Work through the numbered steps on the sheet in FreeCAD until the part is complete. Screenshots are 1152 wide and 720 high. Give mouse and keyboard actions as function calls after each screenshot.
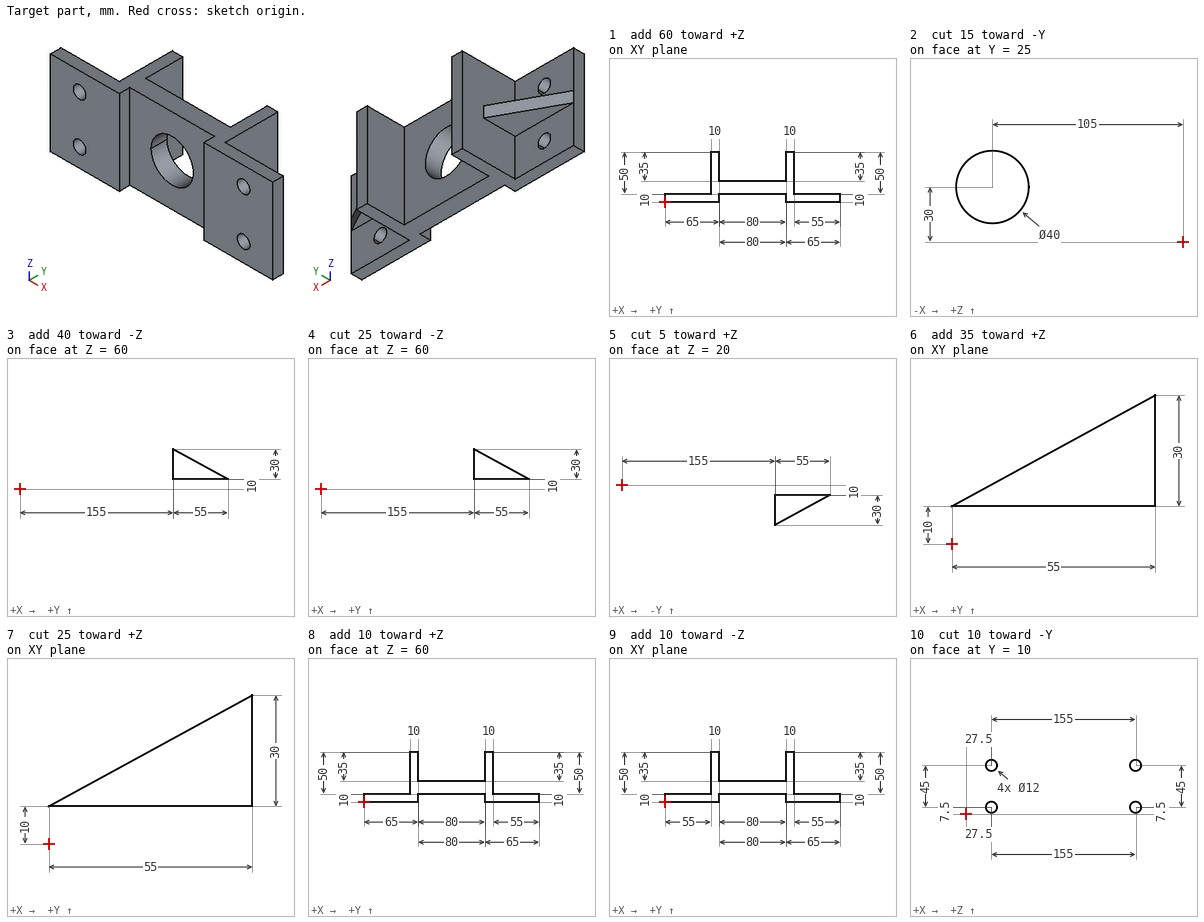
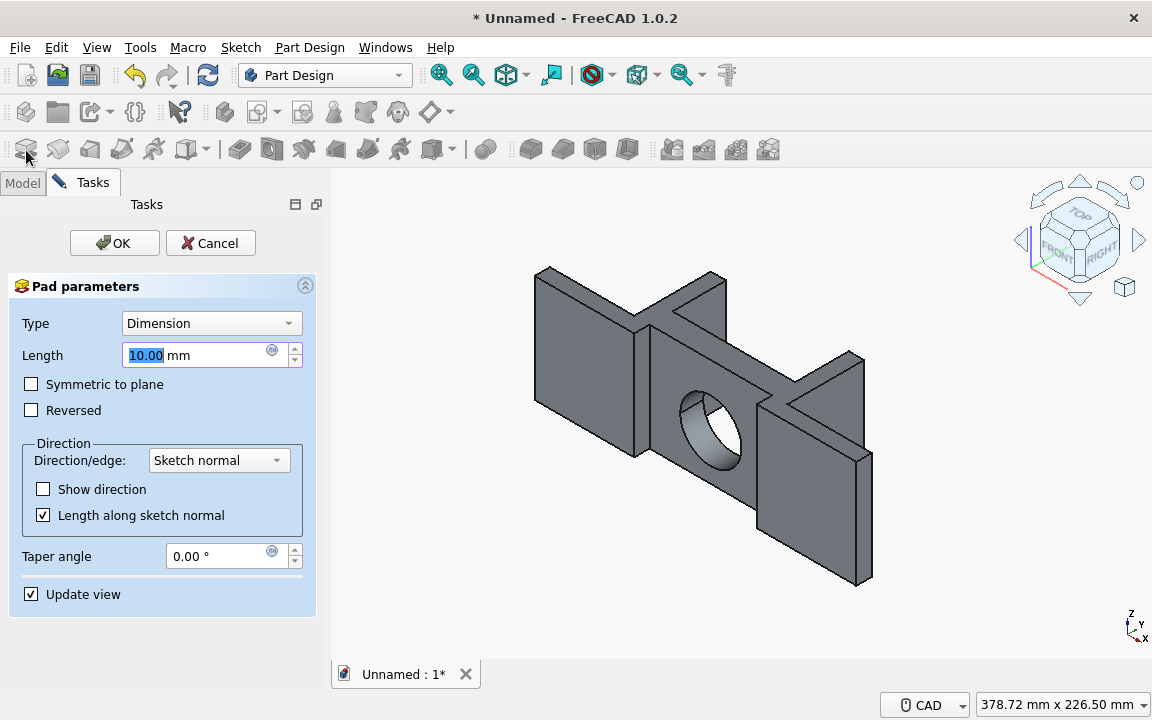
text(10)
key(Tab)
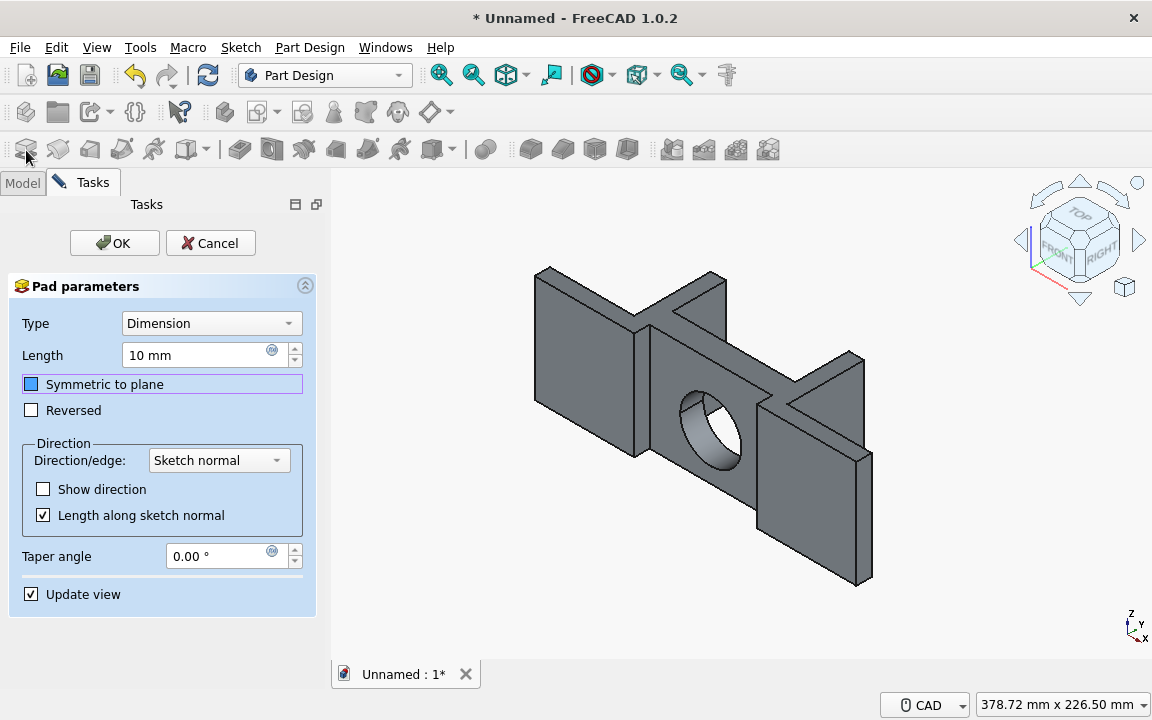
click(30, 410)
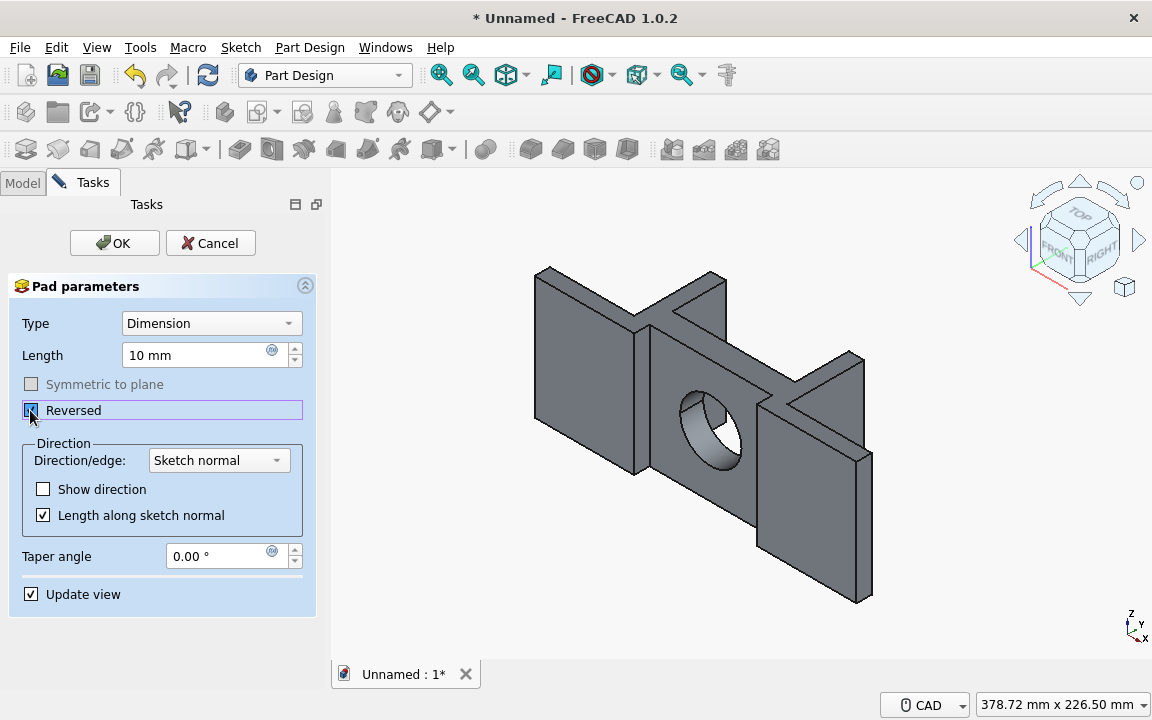
click(115, 243)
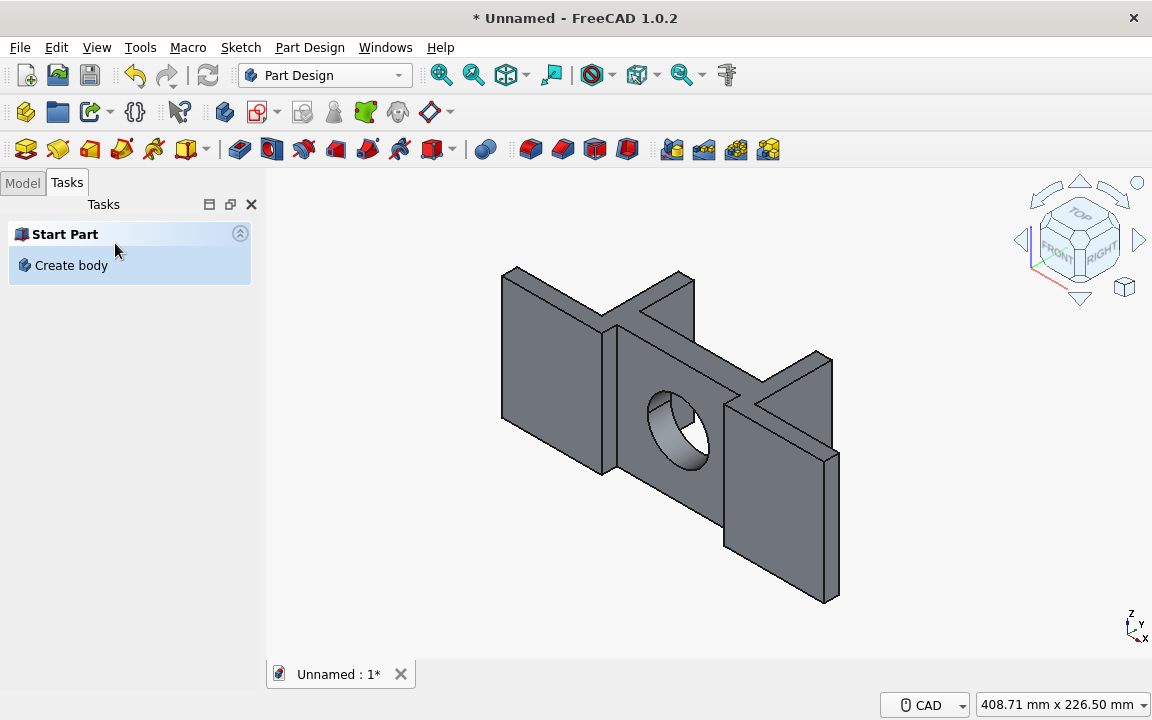
click(713, 410)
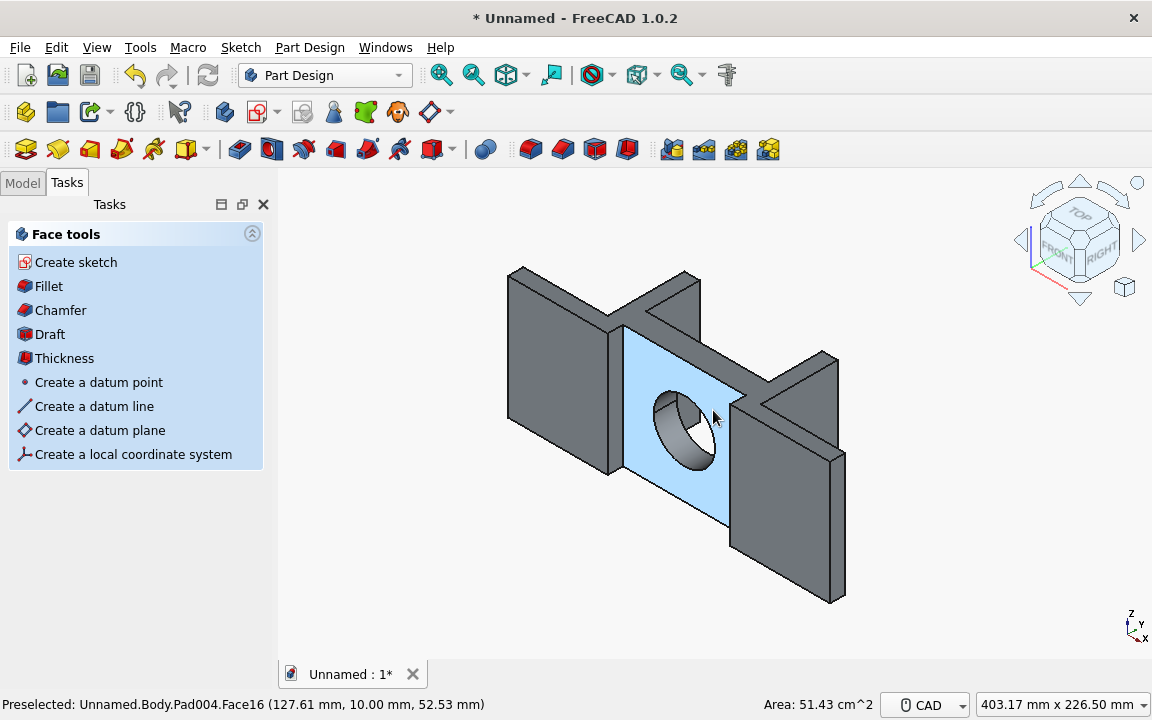
click(258, 112)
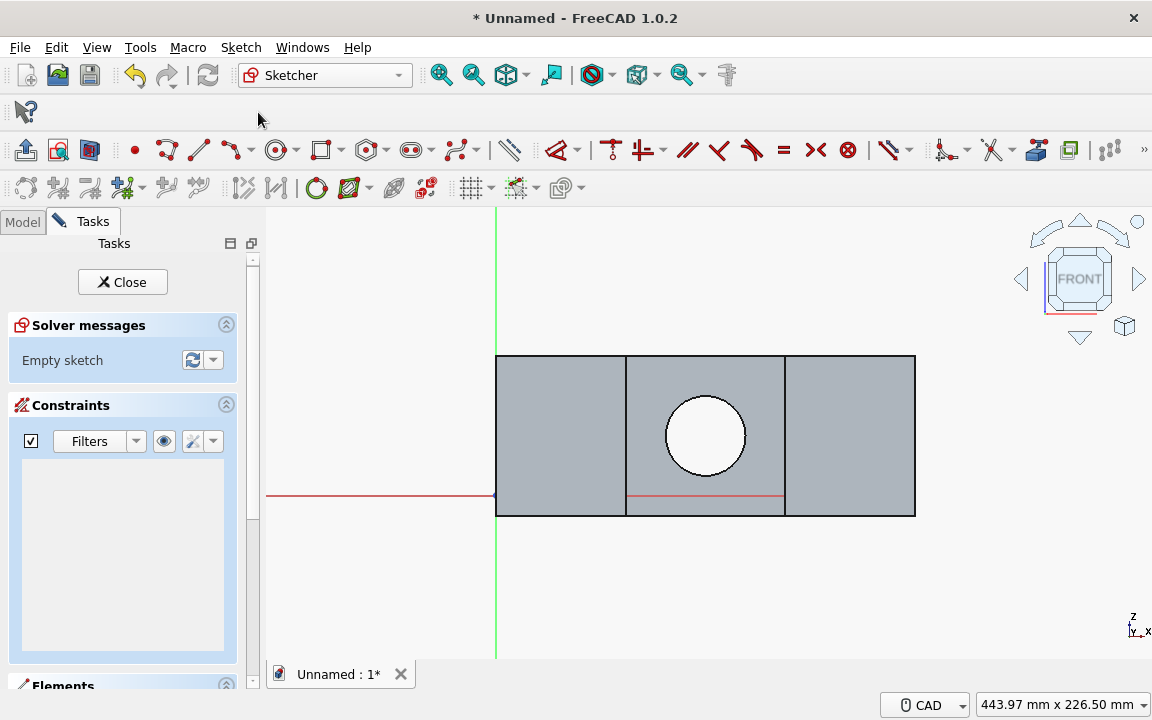
click(276, 150)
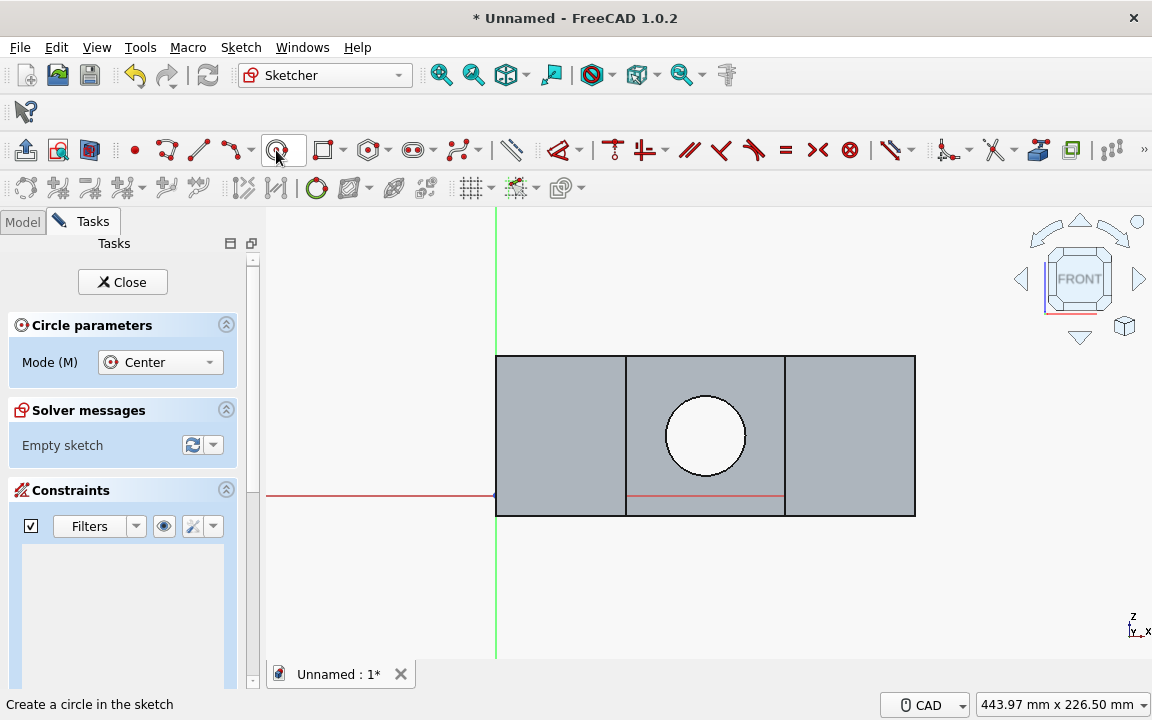
scroll(551, 391, up, 4)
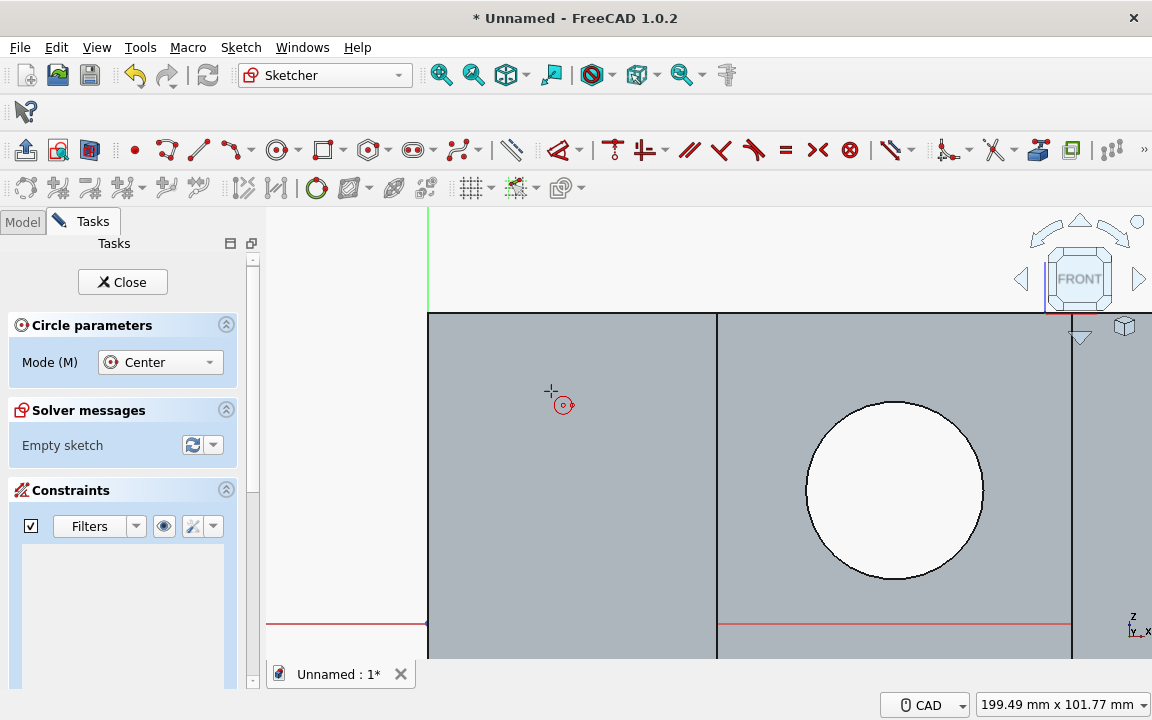
click(551, 391)
move(569, 372)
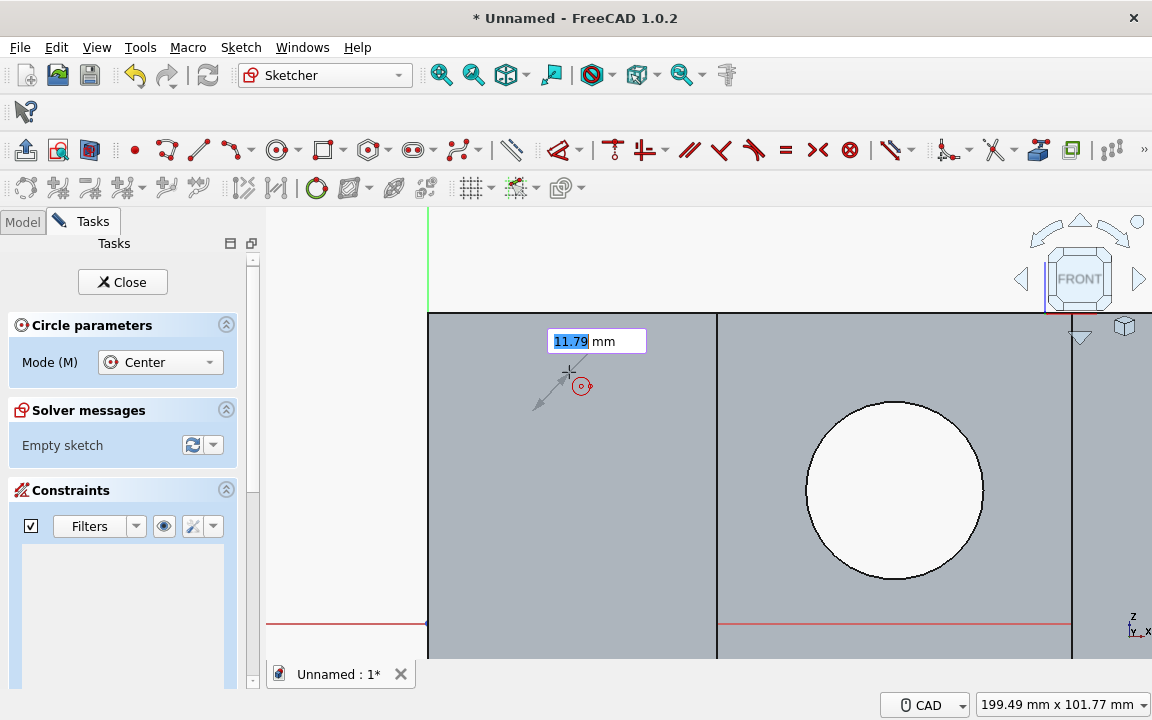
text(12)
key(Return)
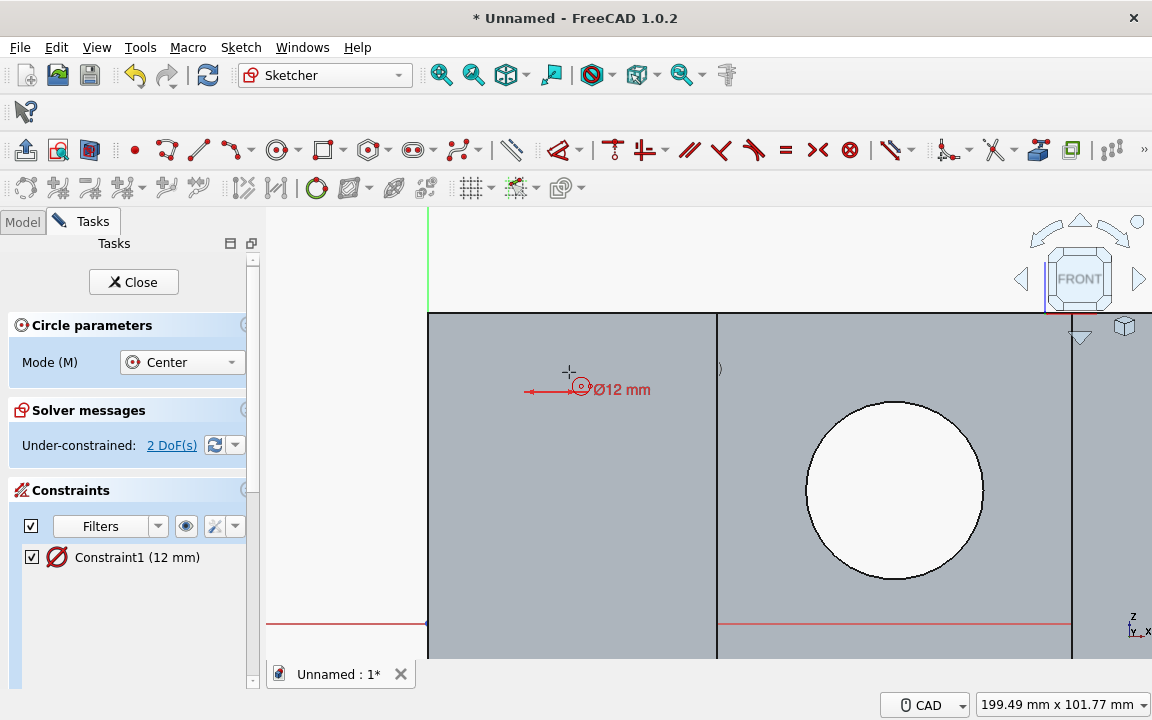
click(551, 591)
move(569, 572)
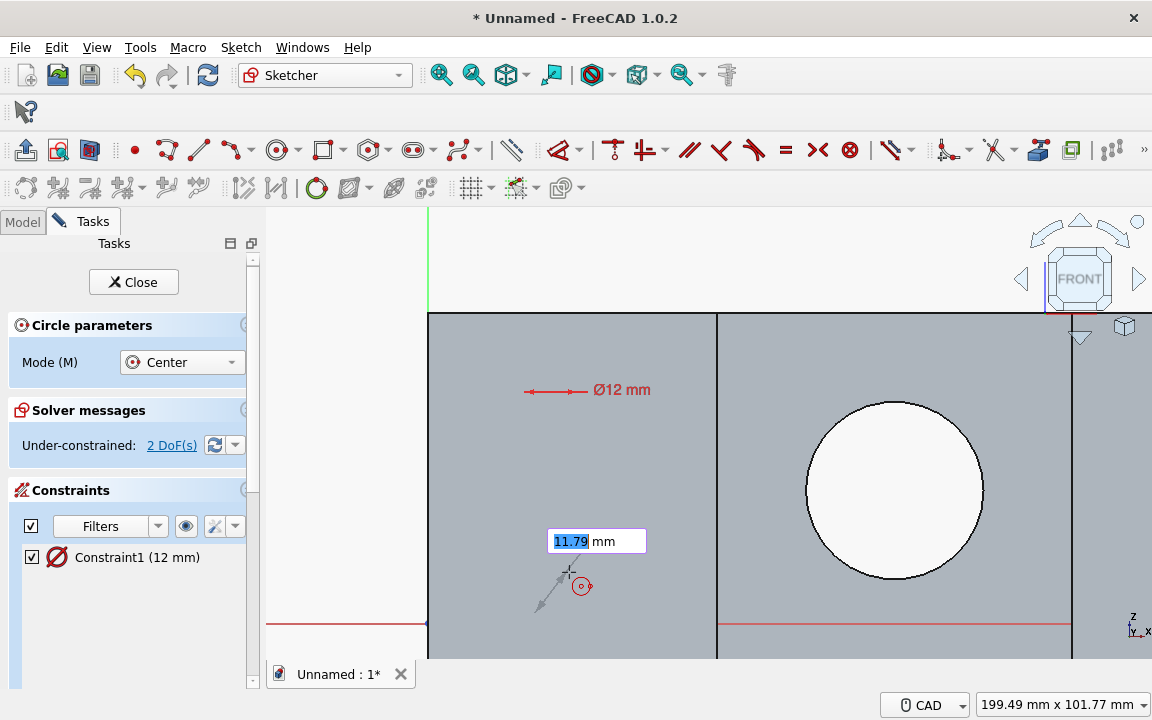
text(12)
key(Return)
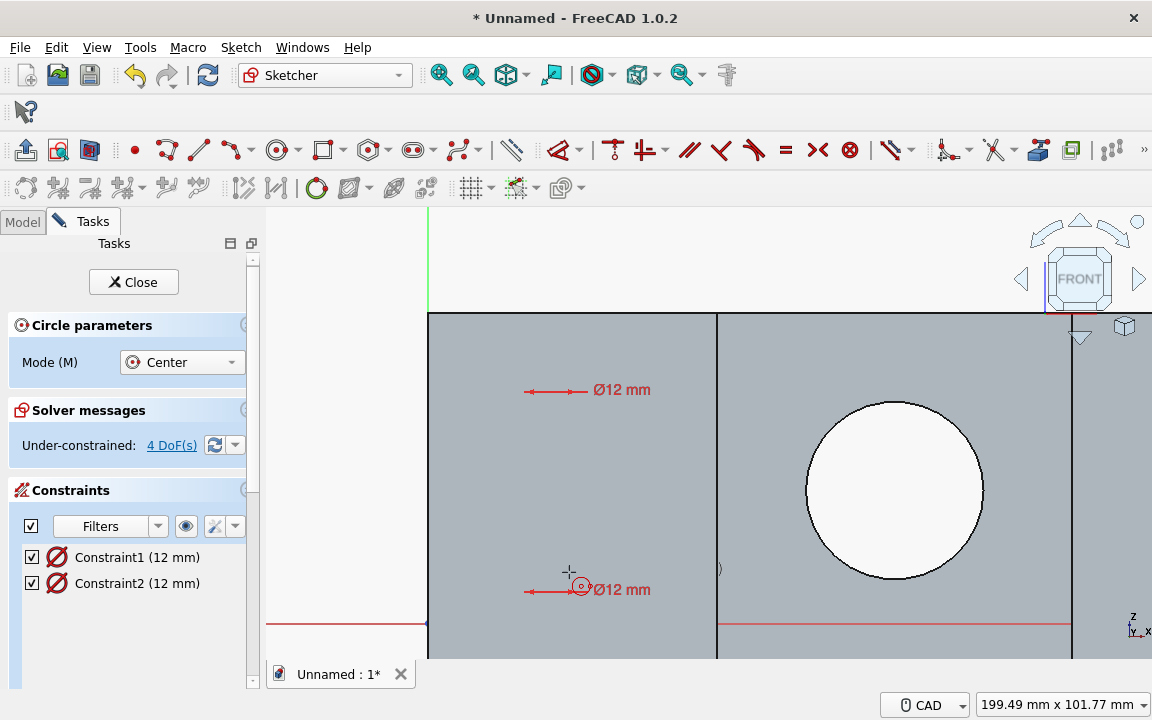
scroll(389, 359, down, 3)